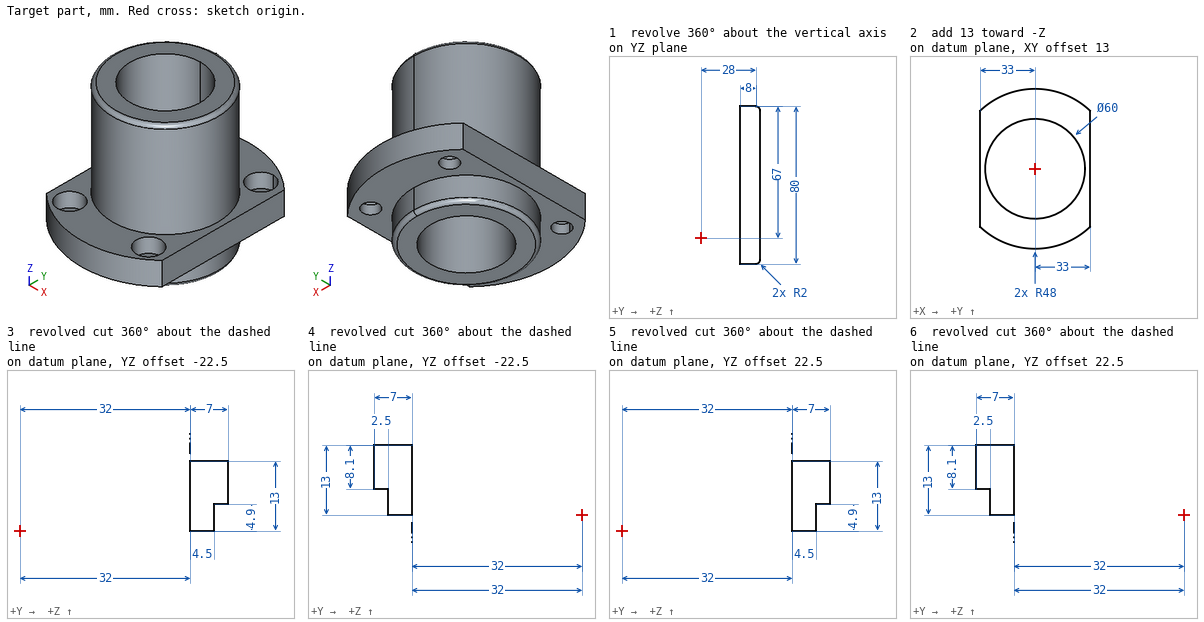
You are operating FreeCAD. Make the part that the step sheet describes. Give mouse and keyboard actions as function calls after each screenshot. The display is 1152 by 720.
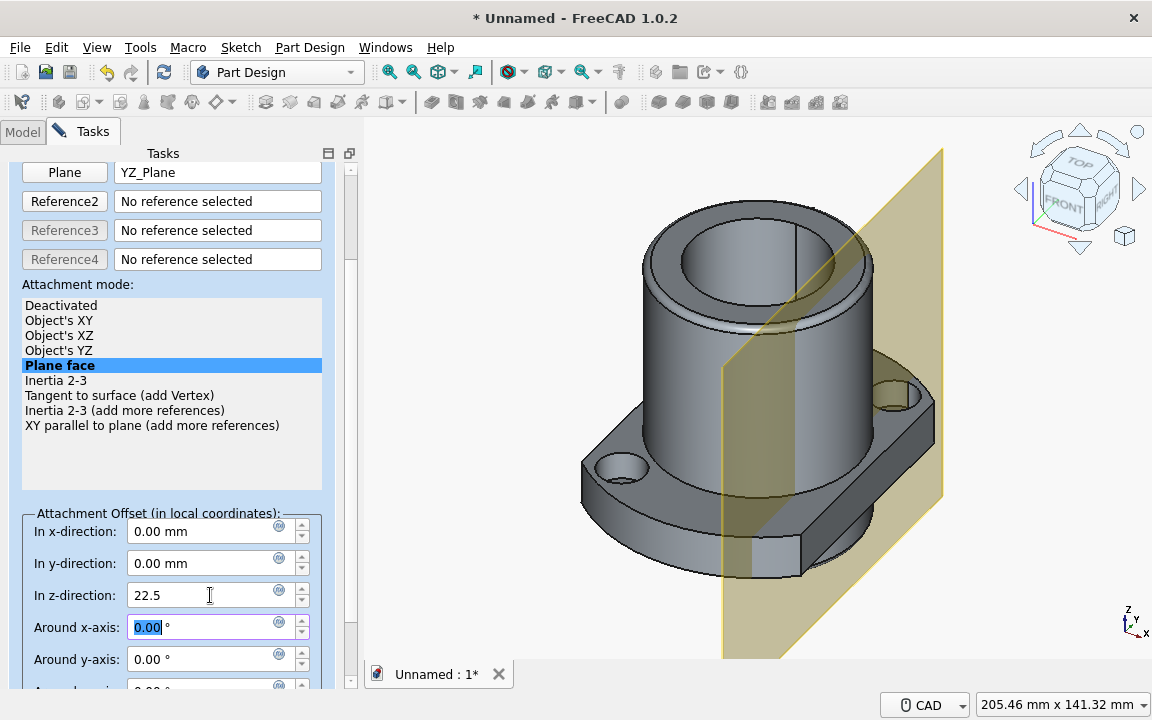
scroll(351, 426, up, 3)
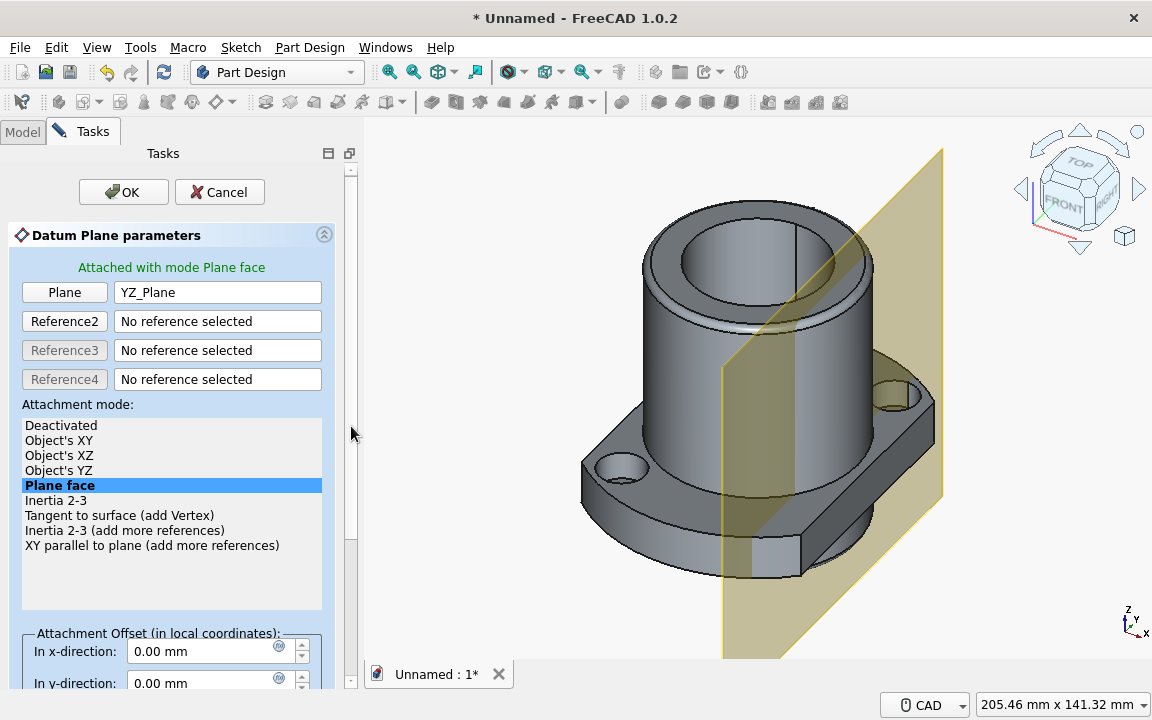
click(124, 192)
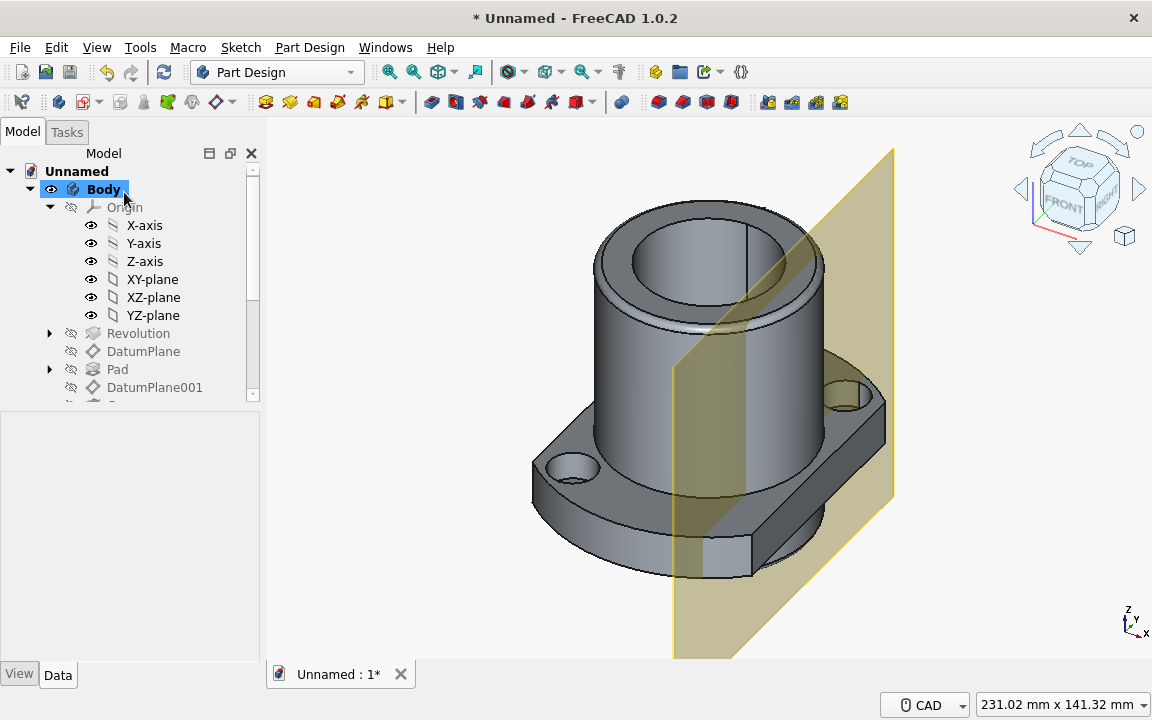
scroll(100, 275, down, 3)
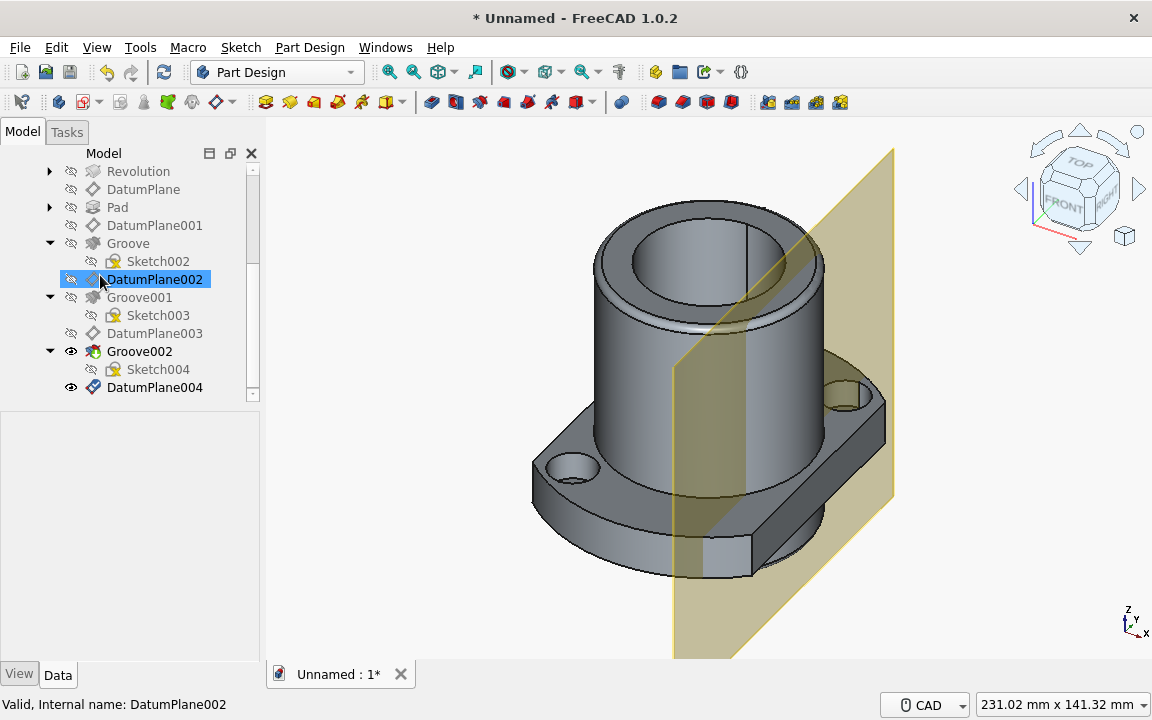
click(116, 387)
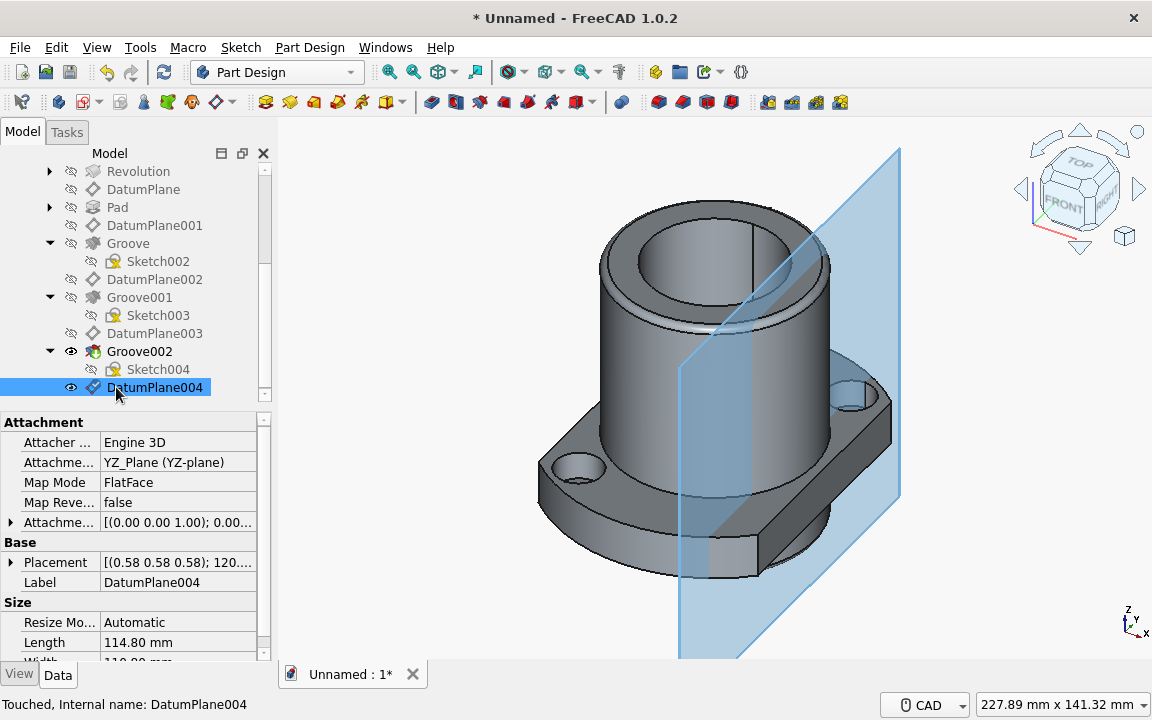
click(84, 102)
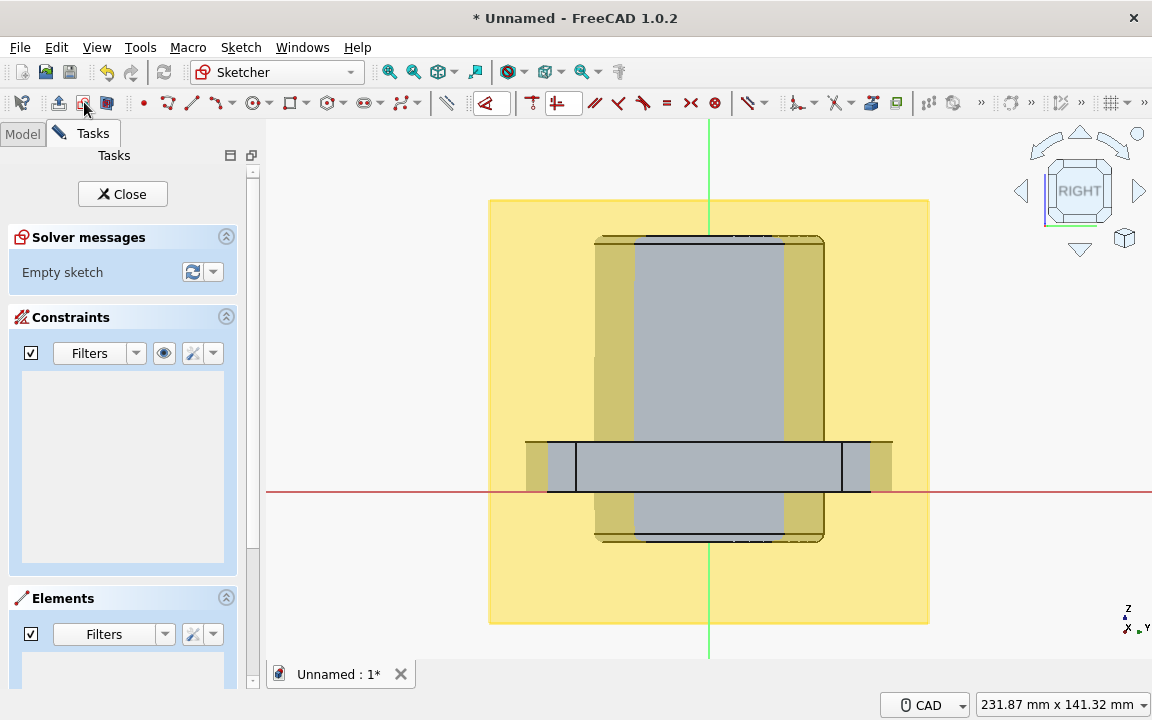
click(108, 104)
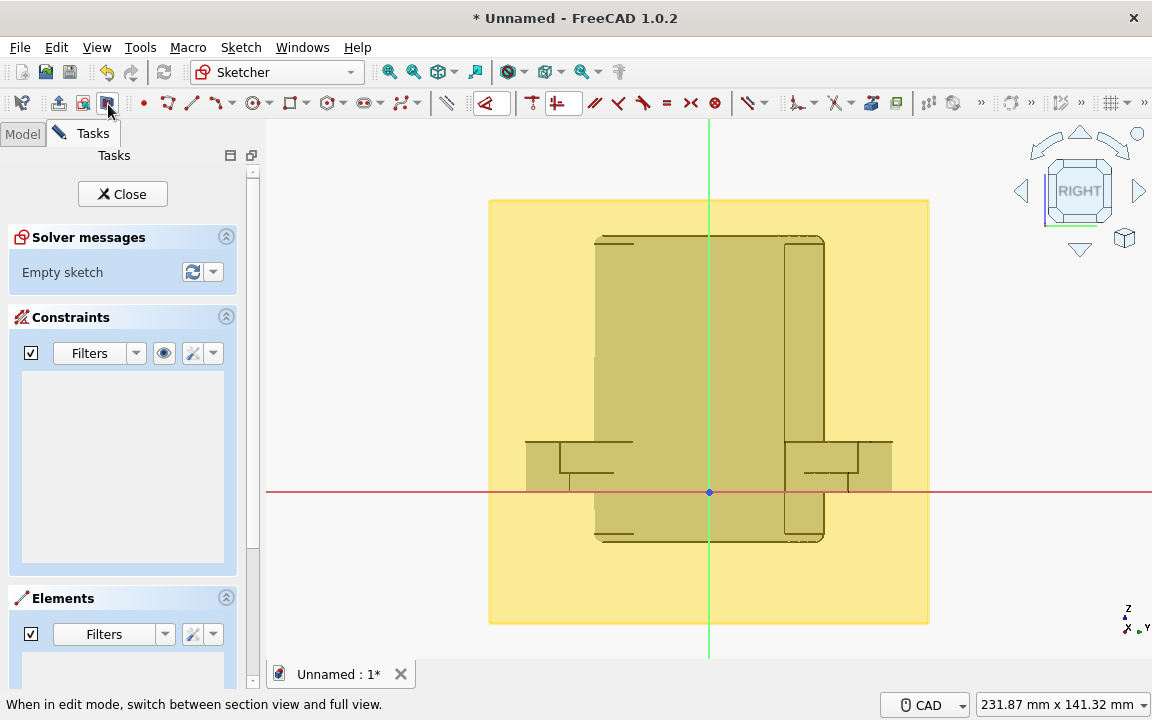
scroll(632, 515, up, 6)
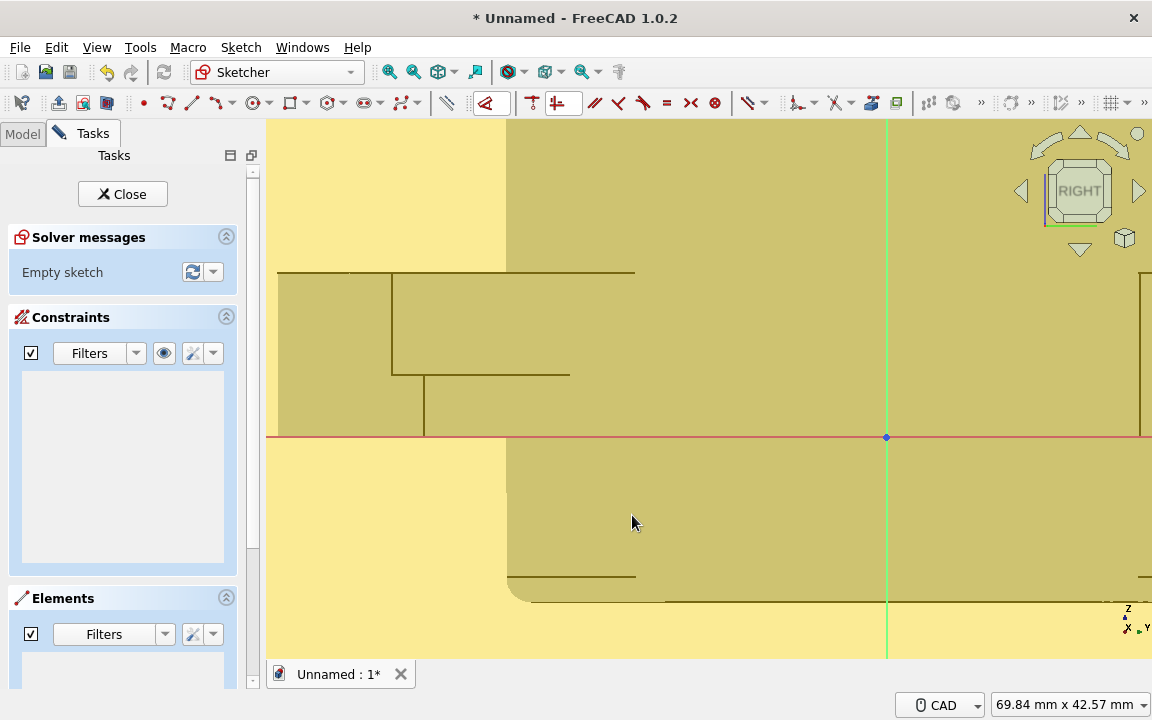
click(168, 104)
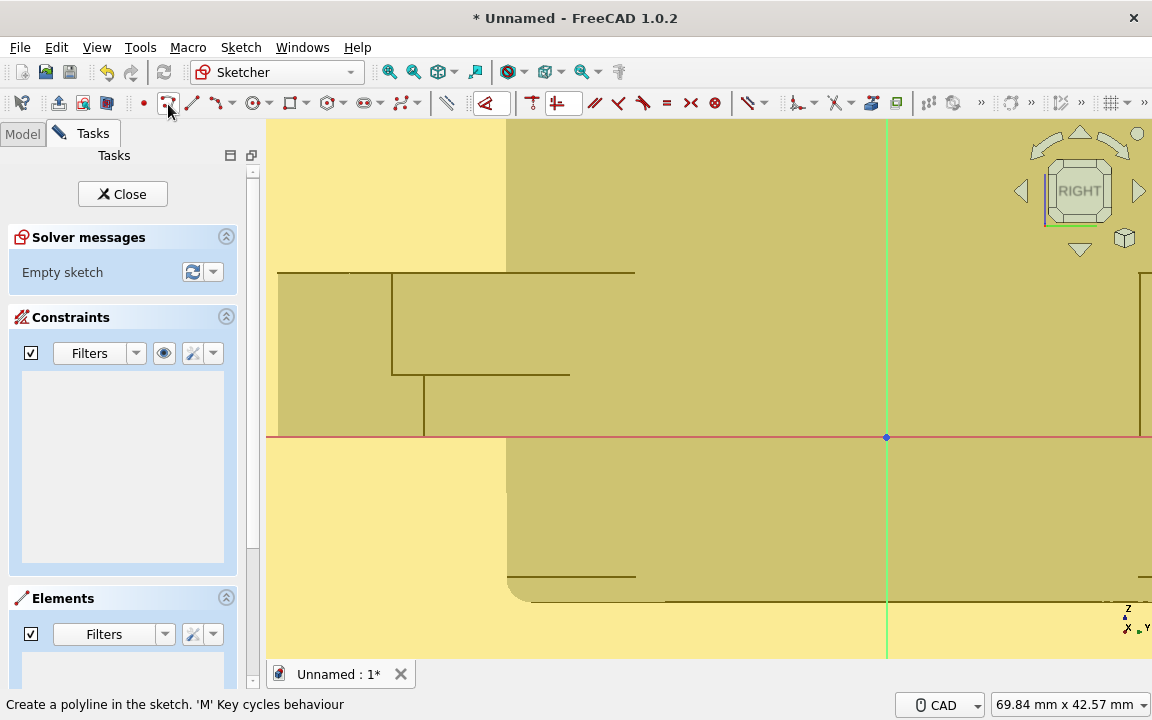
click(481, 437)
click(481, 273)
click(392, 273)
click(392, 375)
click(424, 375)
click(424, 428)
click(481, 437)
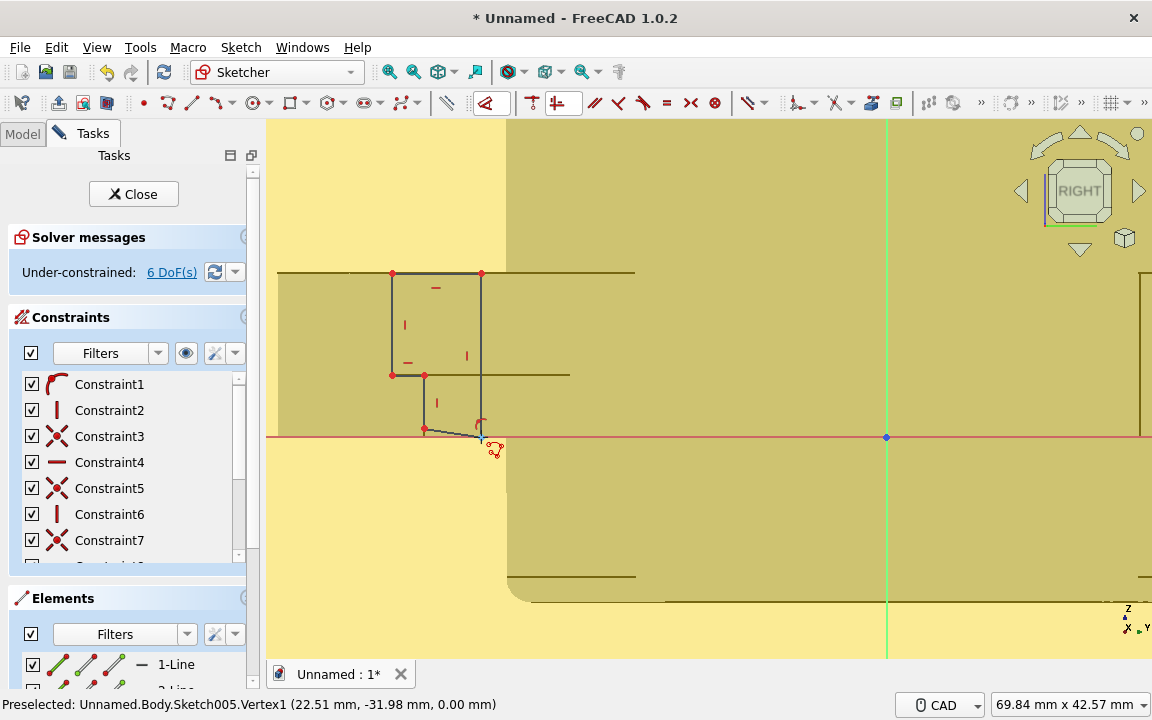
click(192, 104)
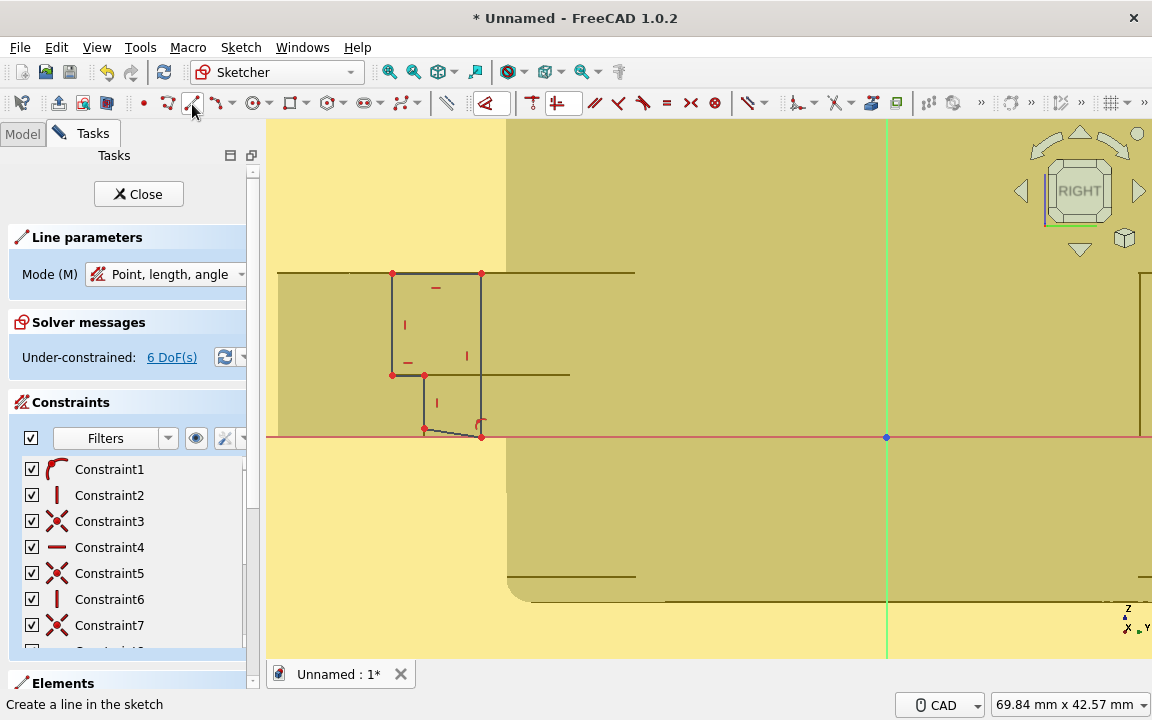
click(481, 454)
click(481, 503)
key(Escape)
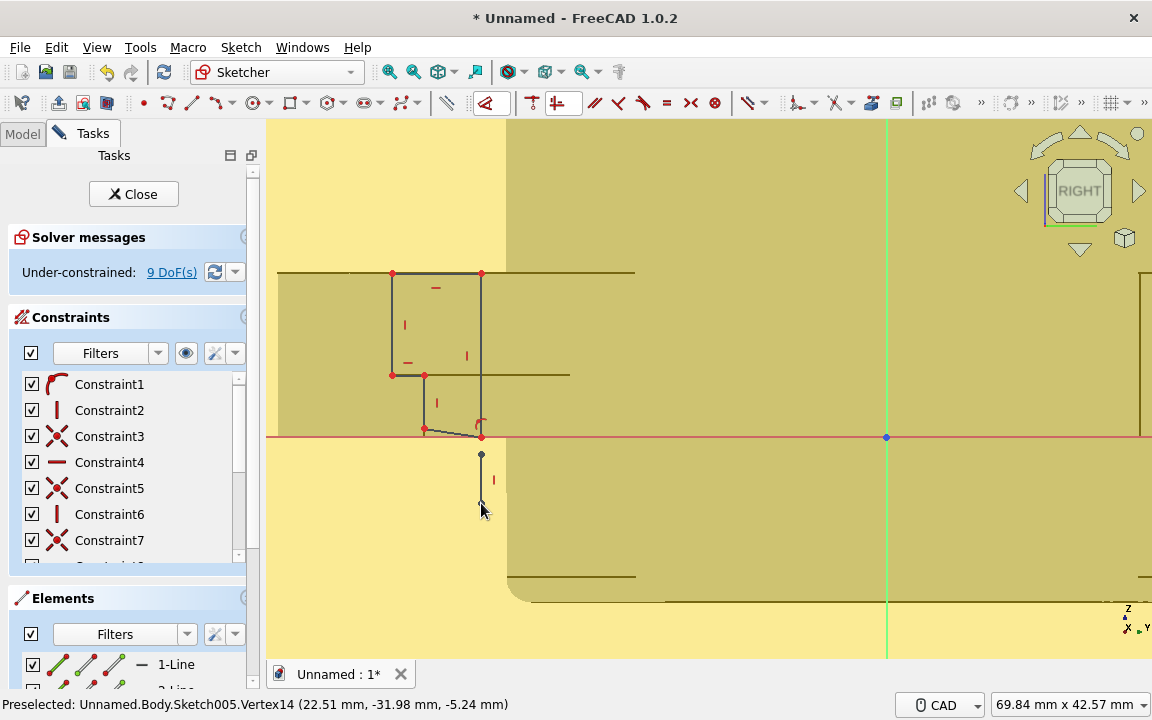
click(481, 470)